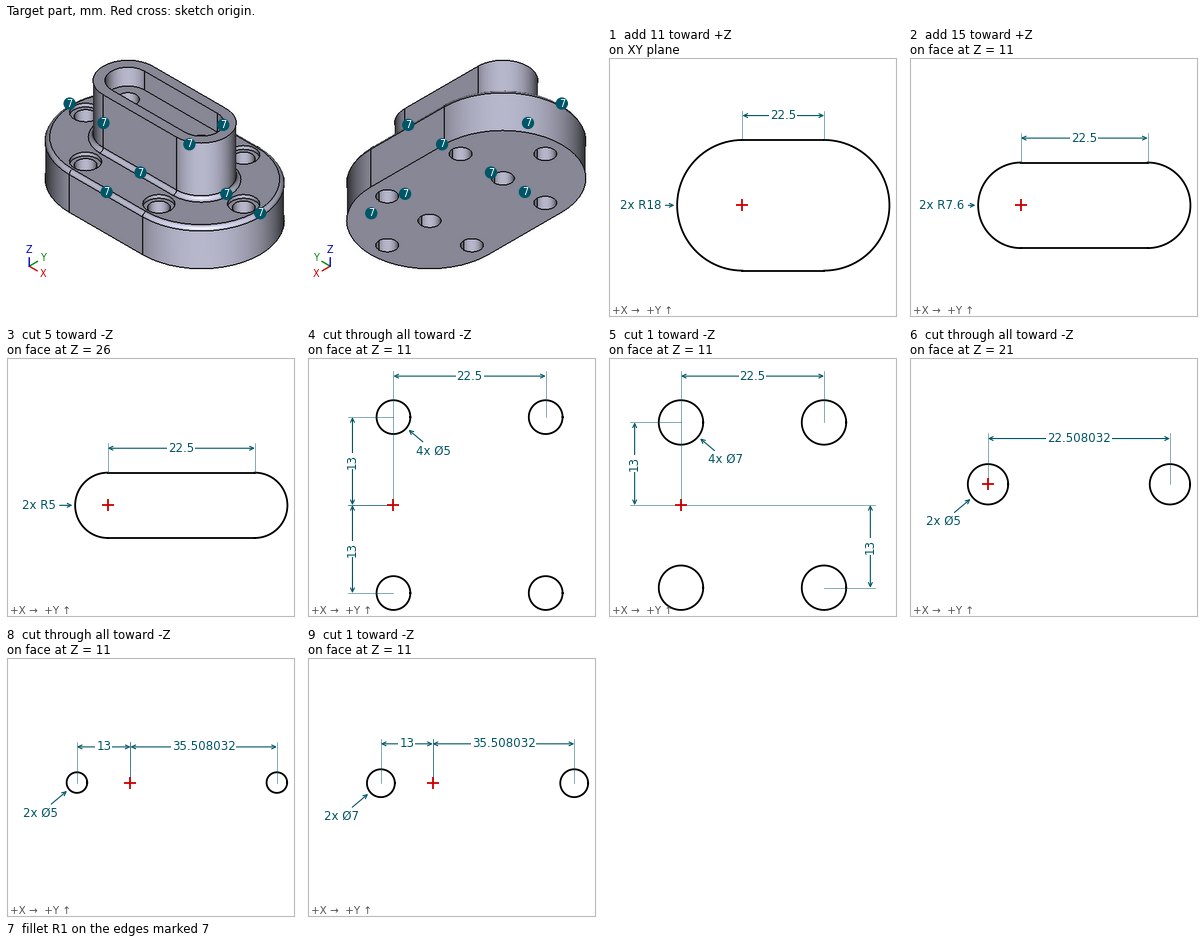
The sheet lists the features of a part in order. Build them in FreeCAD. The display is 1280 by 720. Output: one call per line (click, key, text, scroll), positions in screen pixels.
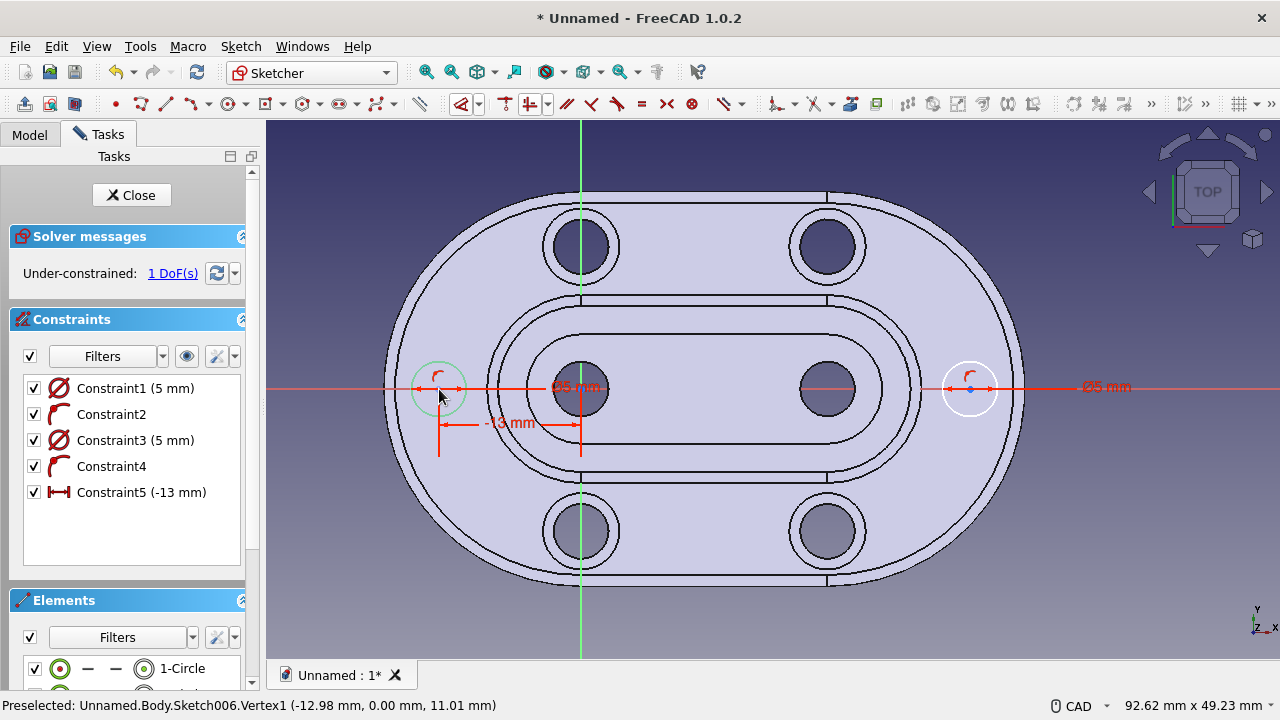
click(970, 389)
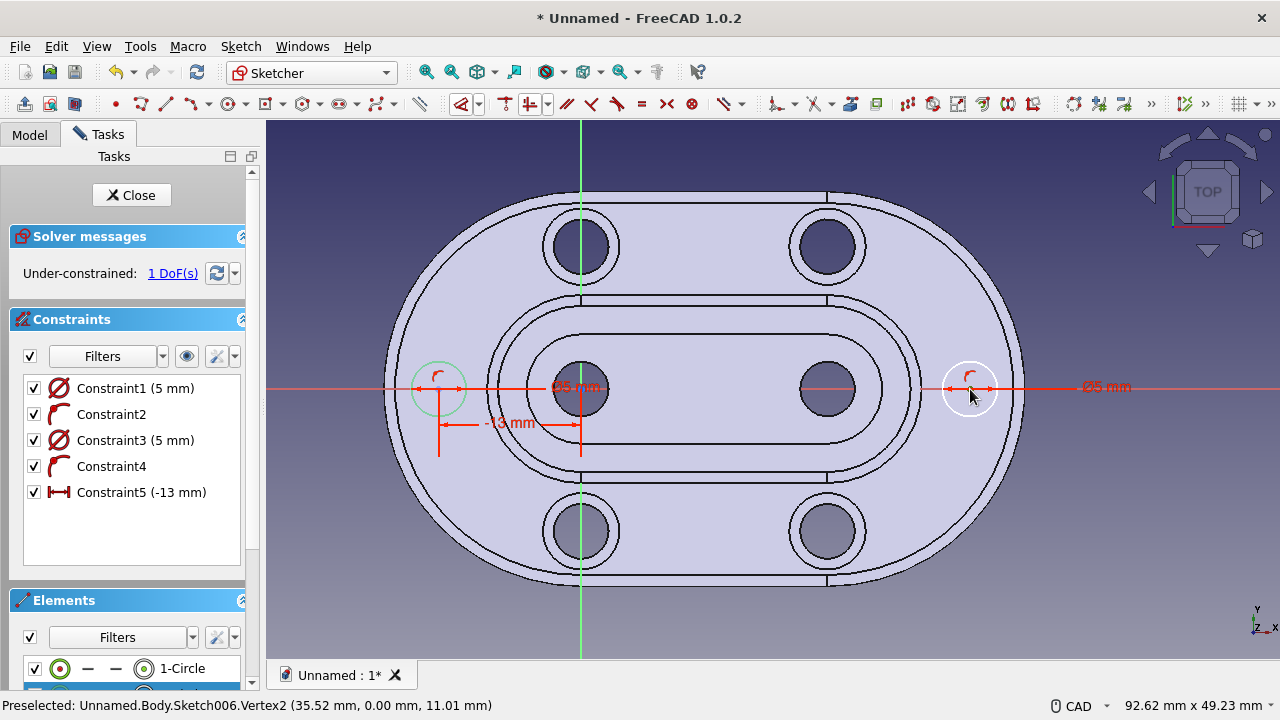
key(l)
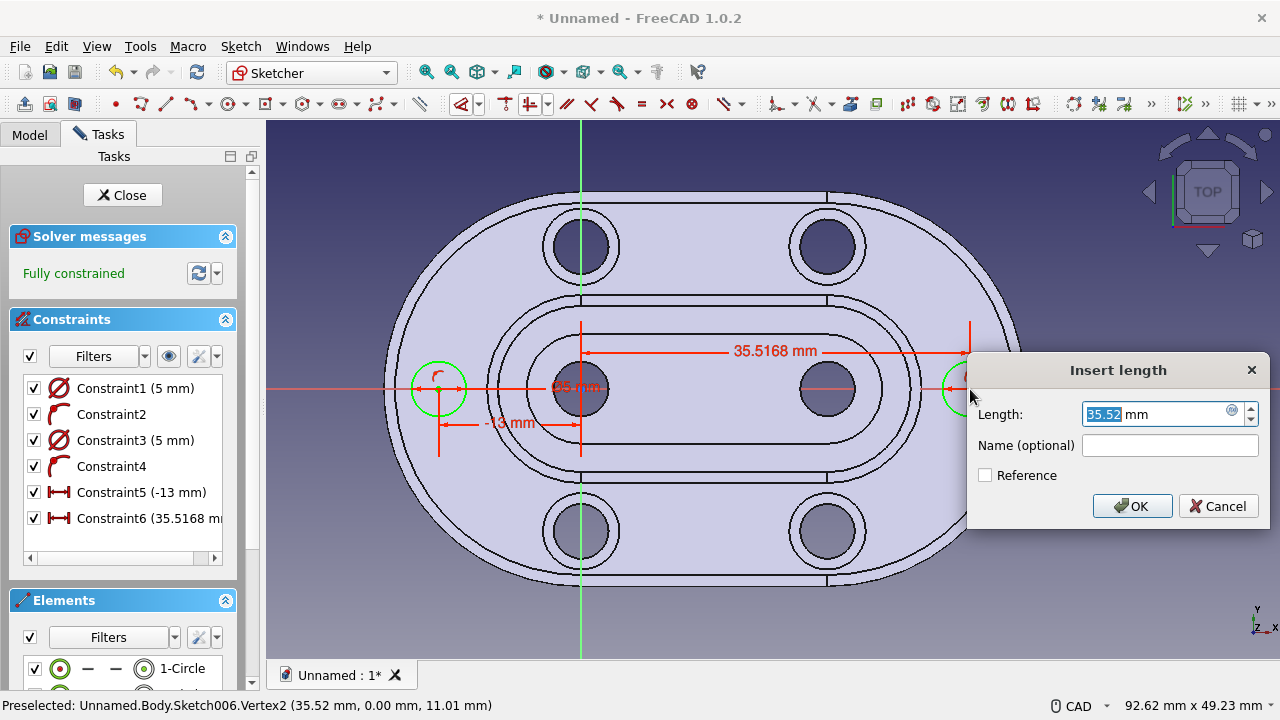
text(35.508032)
key(Return)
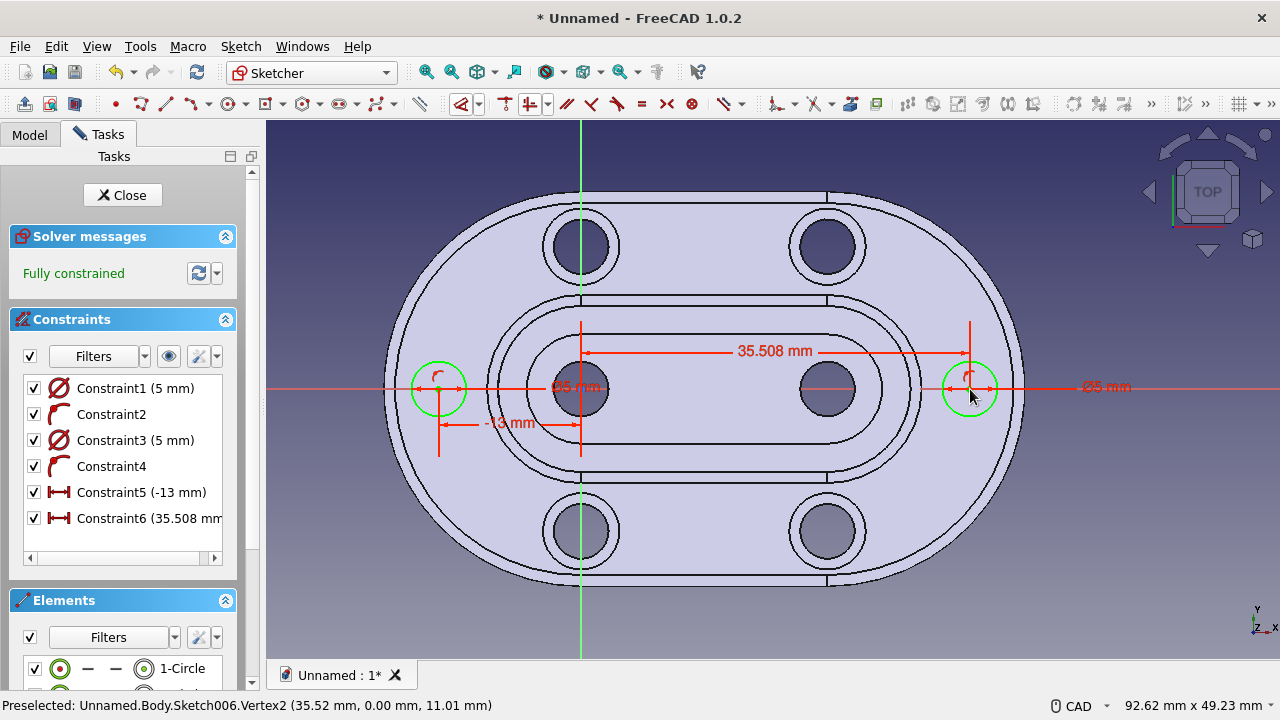
click(123, 195)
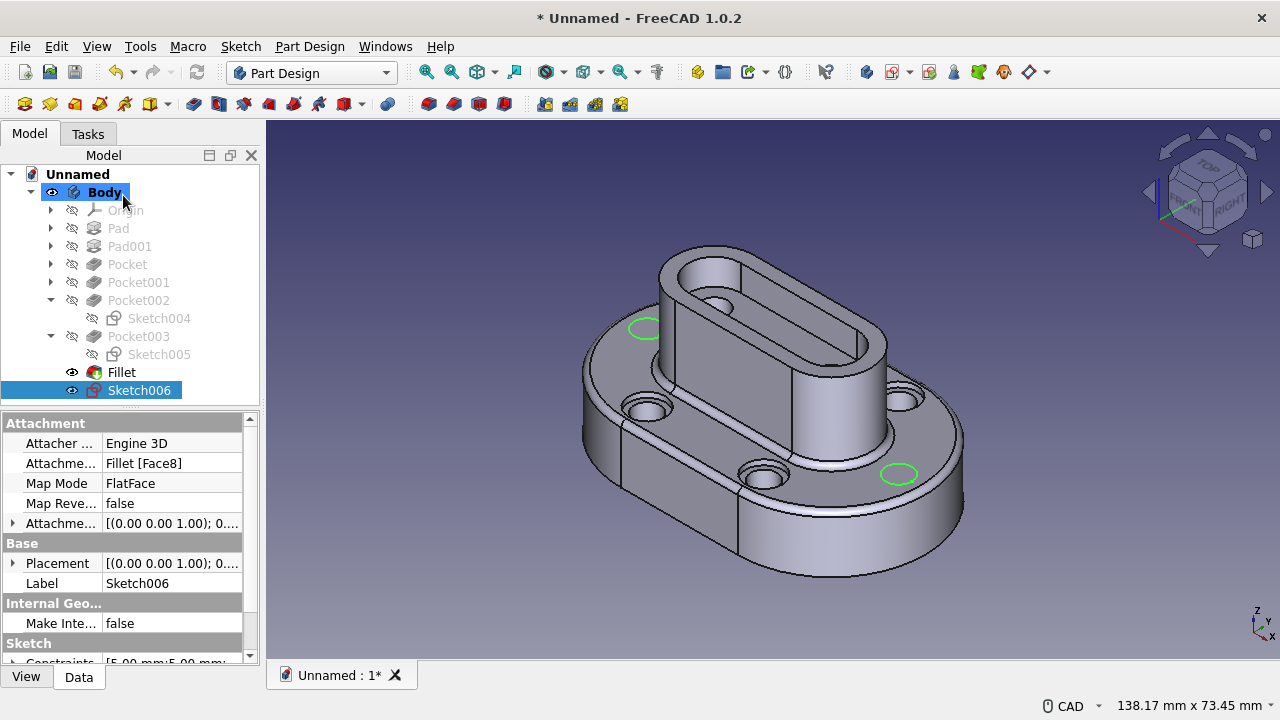
click(194, 104)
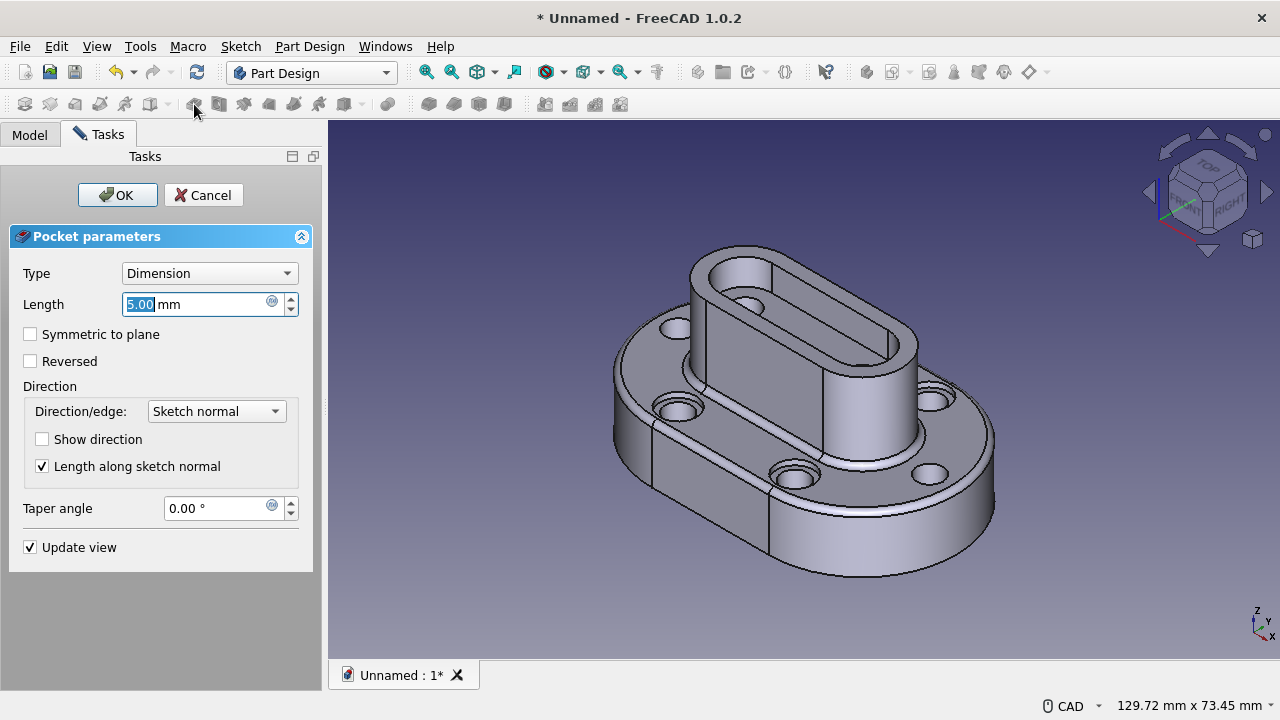
click(210, 274)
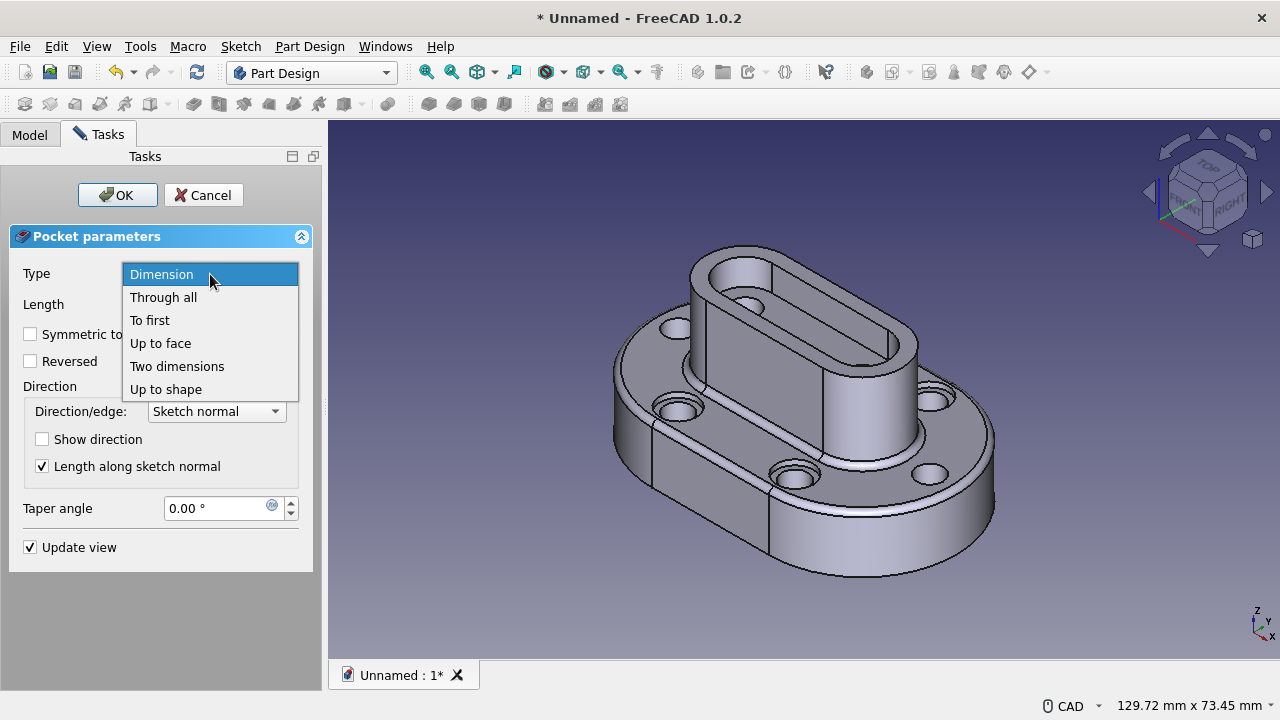
click(208, 298)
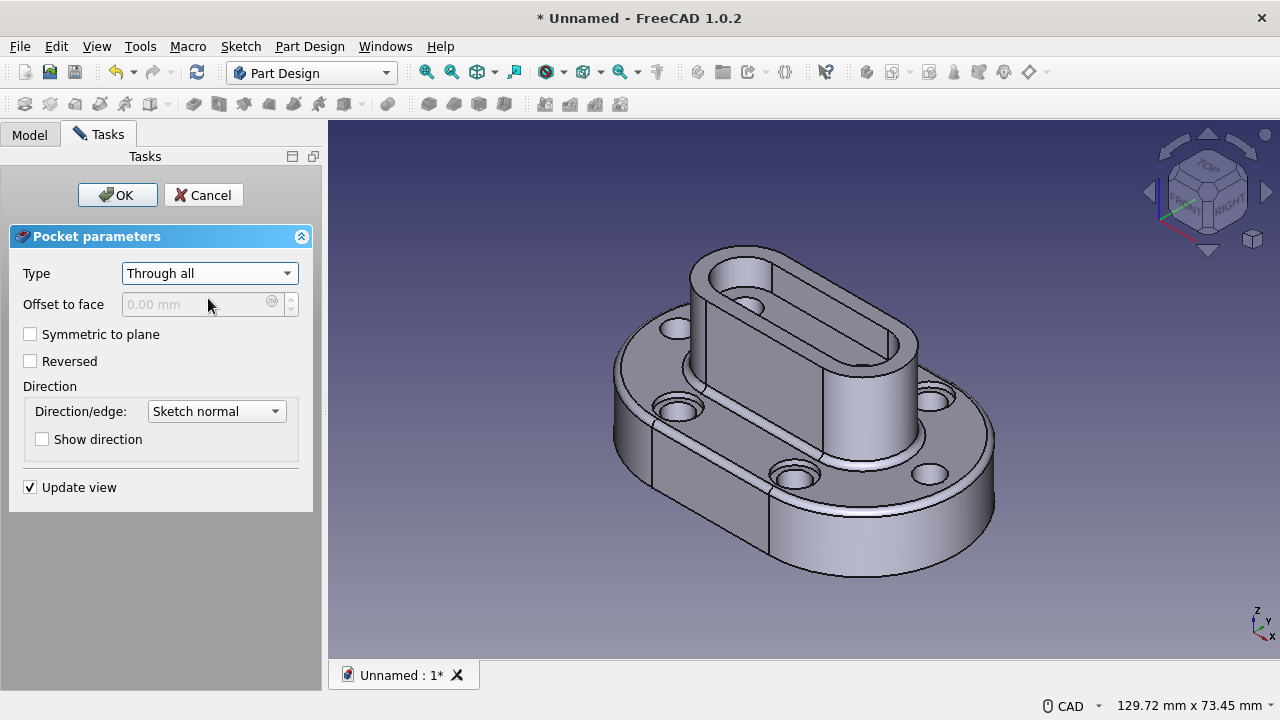
click(118, 195)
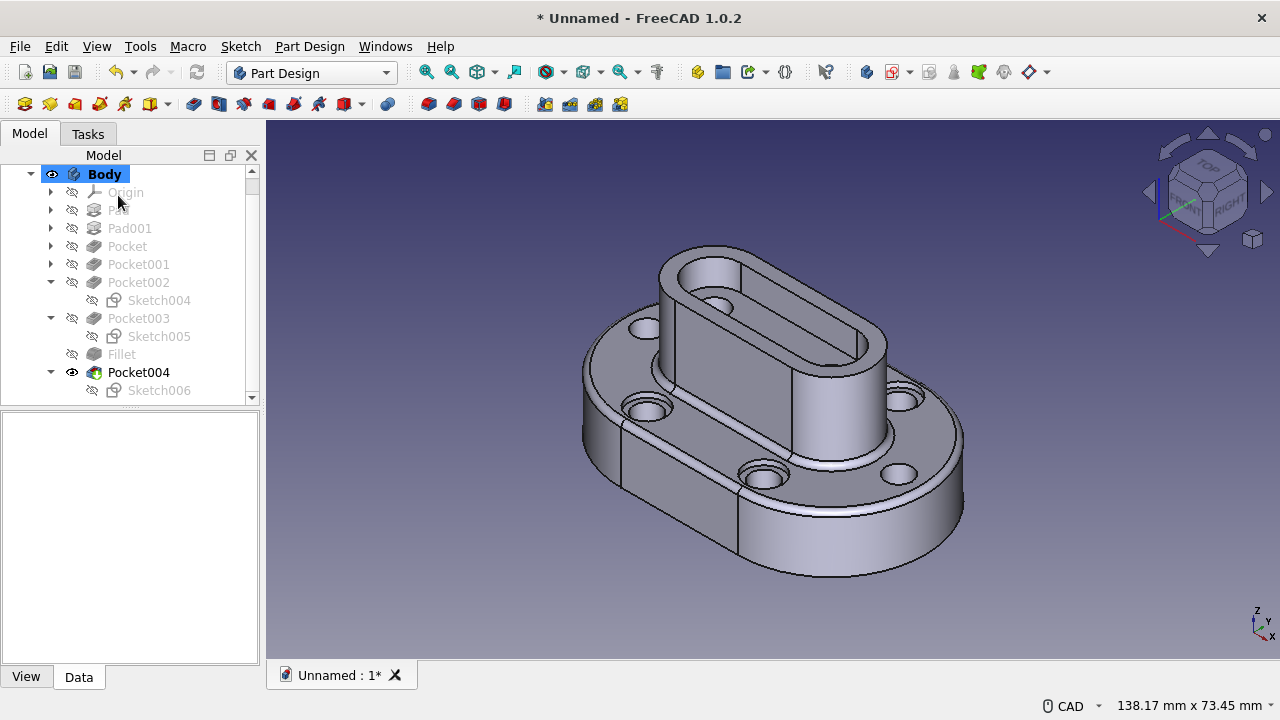
click(697, 444)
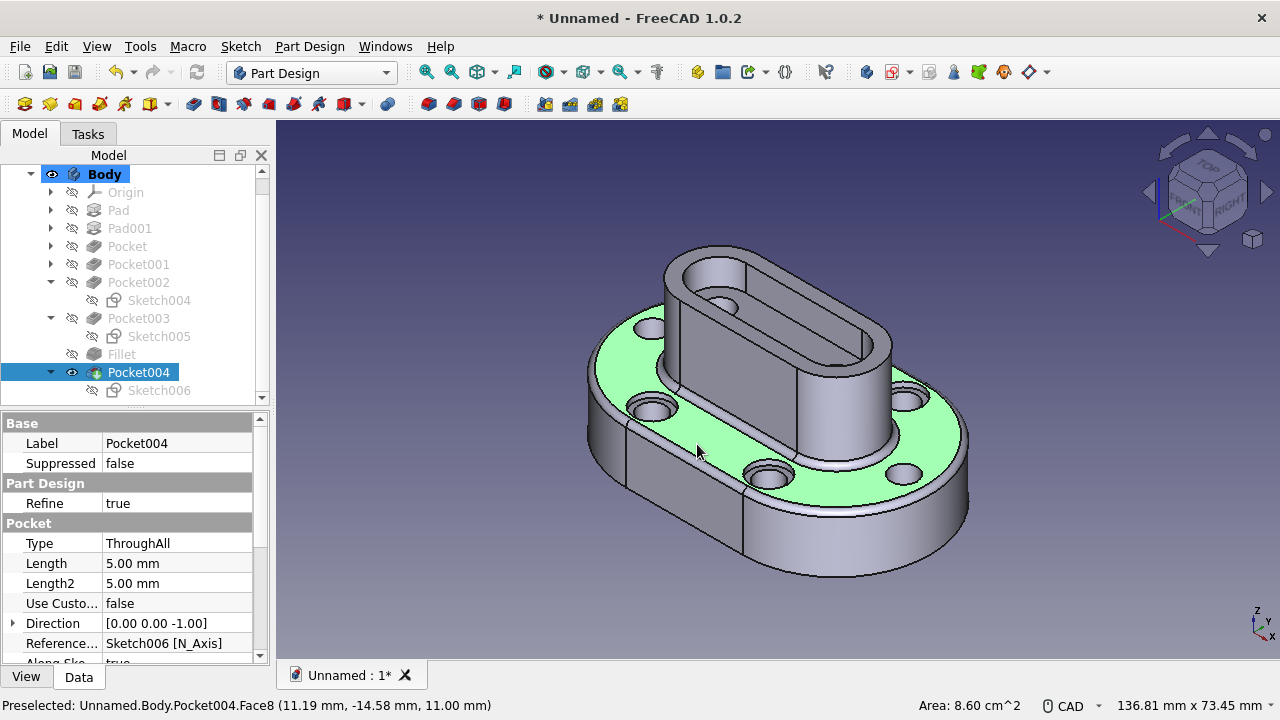
click(892, 72)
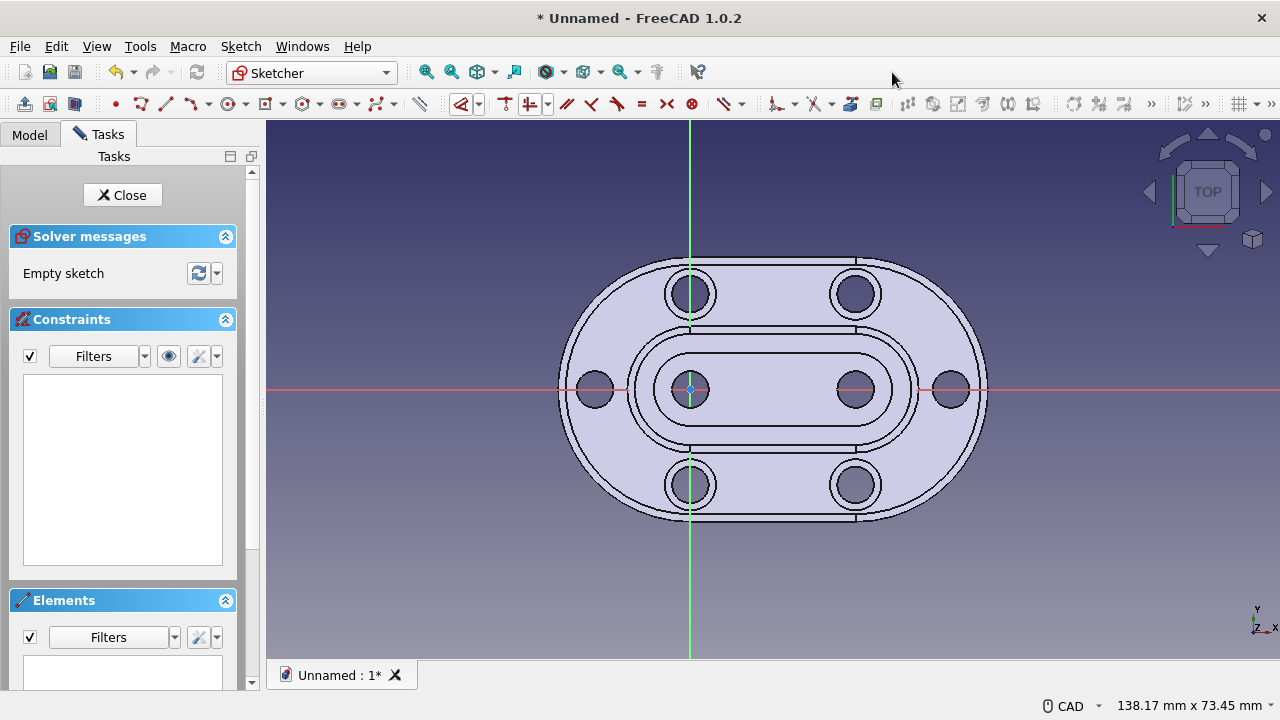
scroll(912, 390, up, 2)